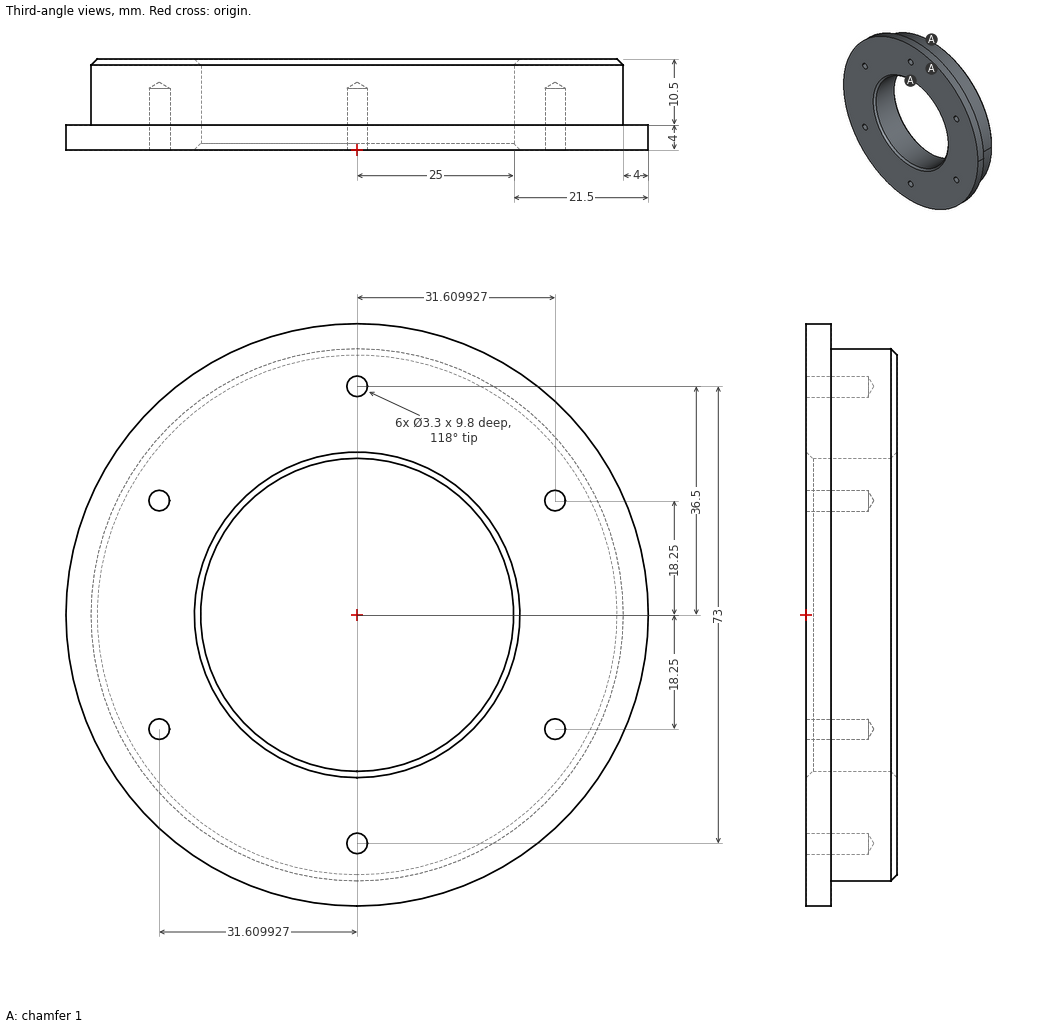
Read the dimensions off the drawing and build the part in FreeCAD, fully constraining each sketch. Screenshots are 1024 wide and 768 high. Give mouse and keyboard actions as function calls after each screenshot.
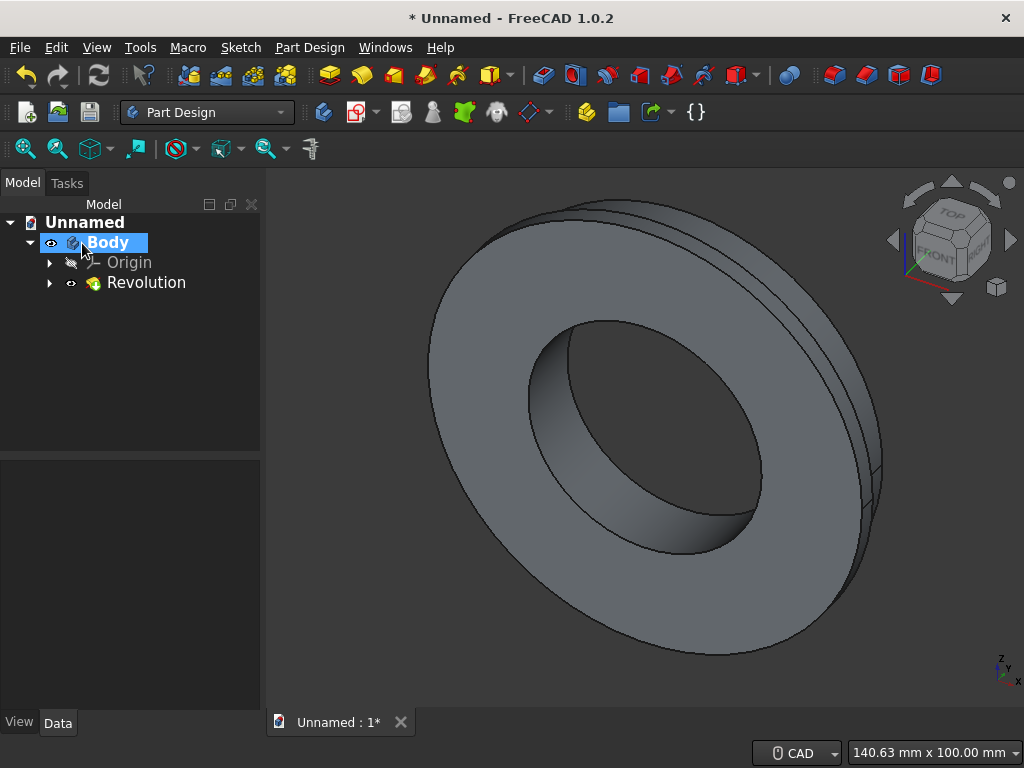
click(26, 150)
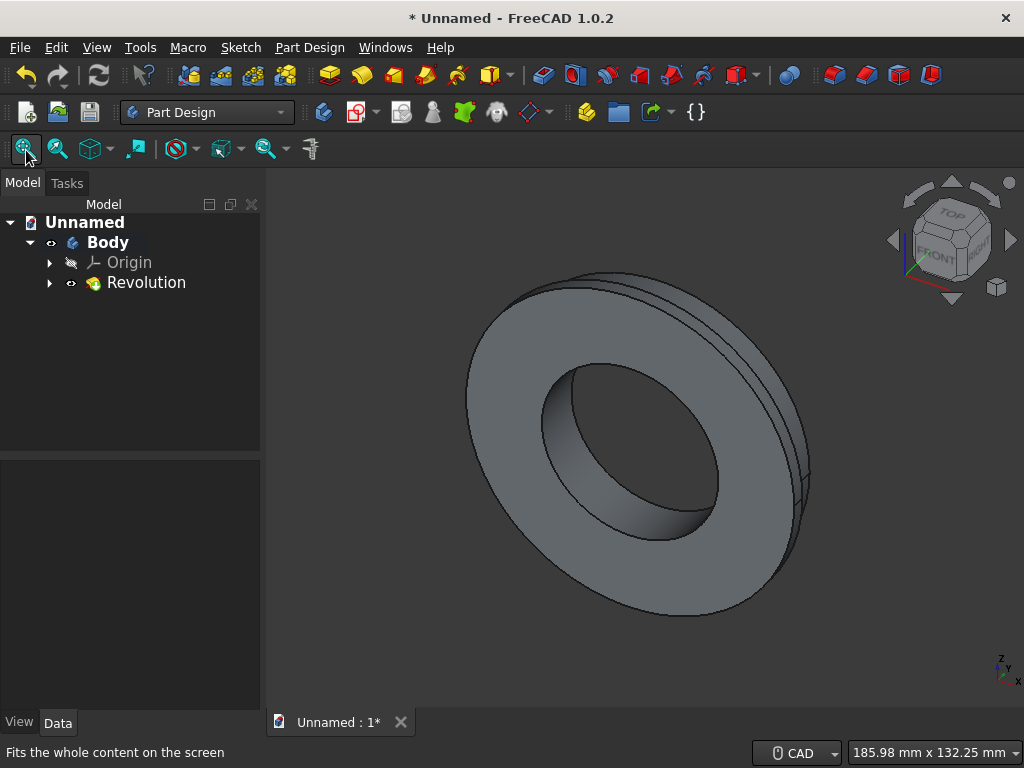
click(536, 509)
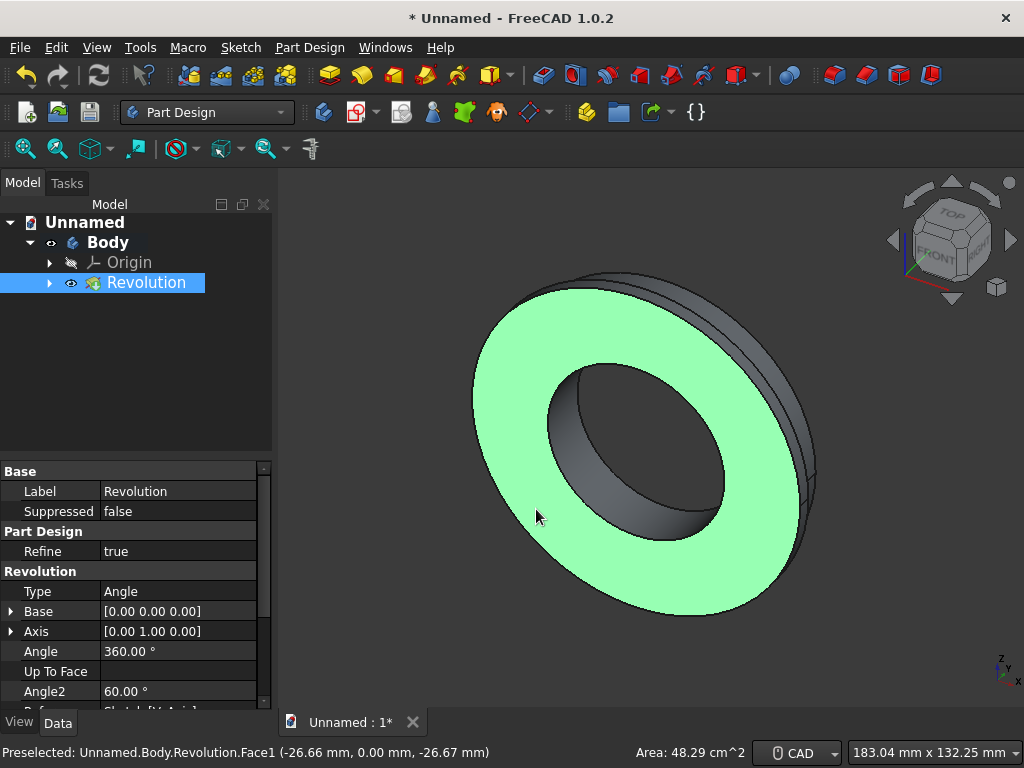
click(356, 112)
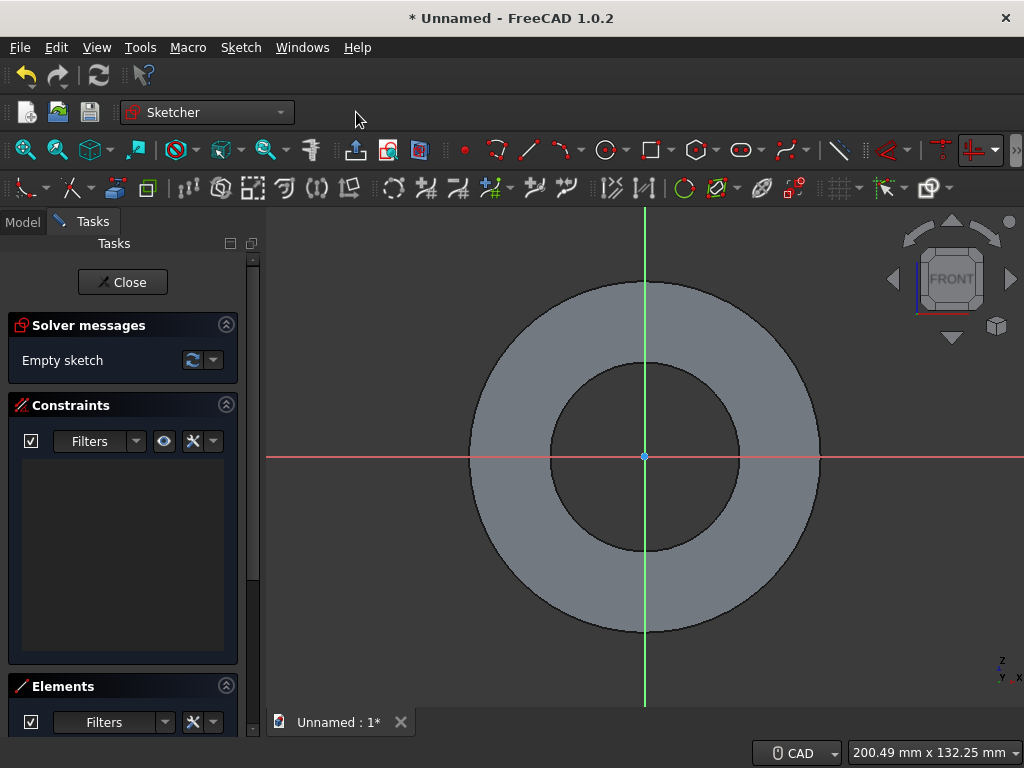
click(606, 150)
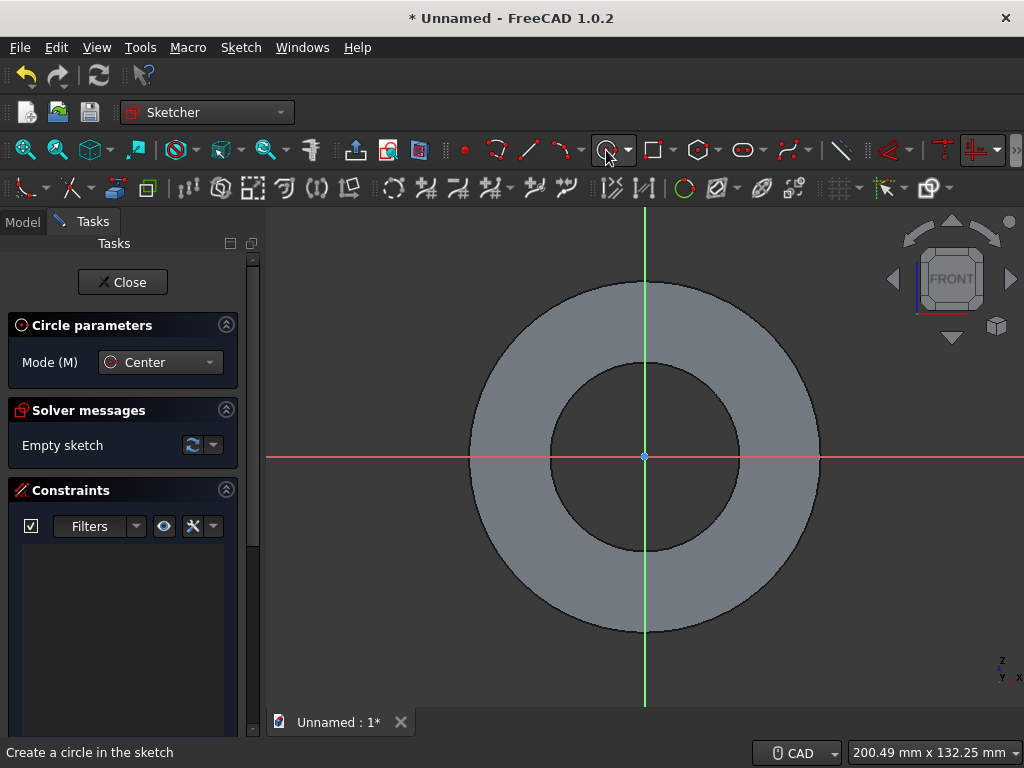
scroll(645, 319, up, 7)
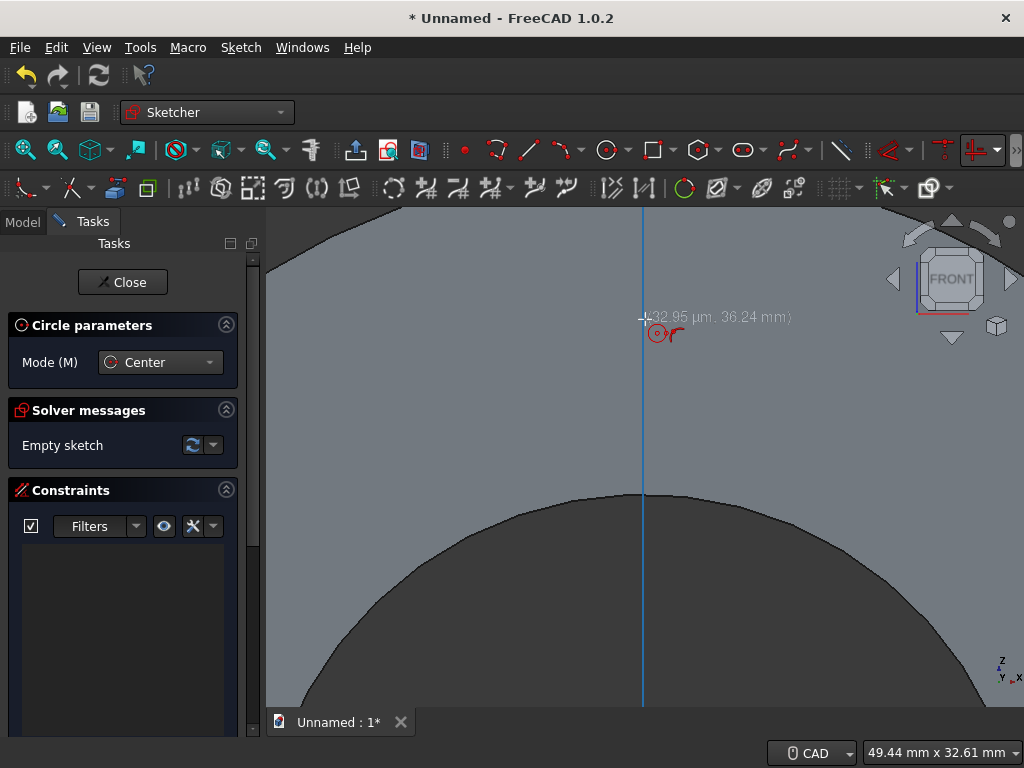
scroll(555, 319, down, 7)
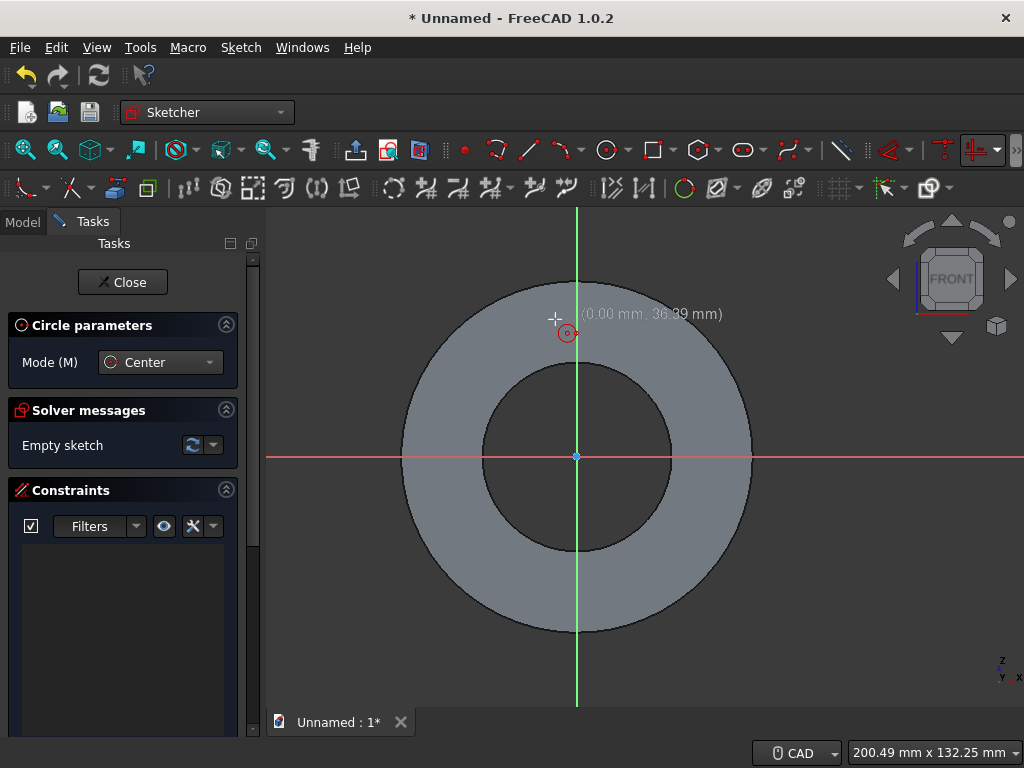
click(577, 319)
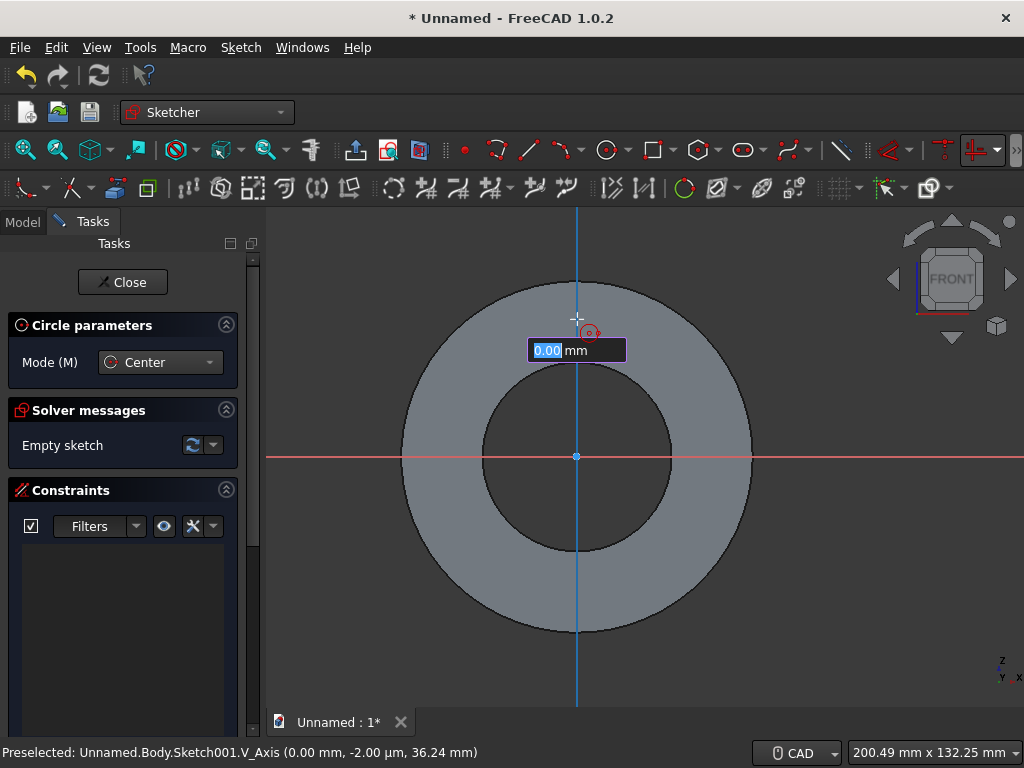
scroll(583, 317, up, 5)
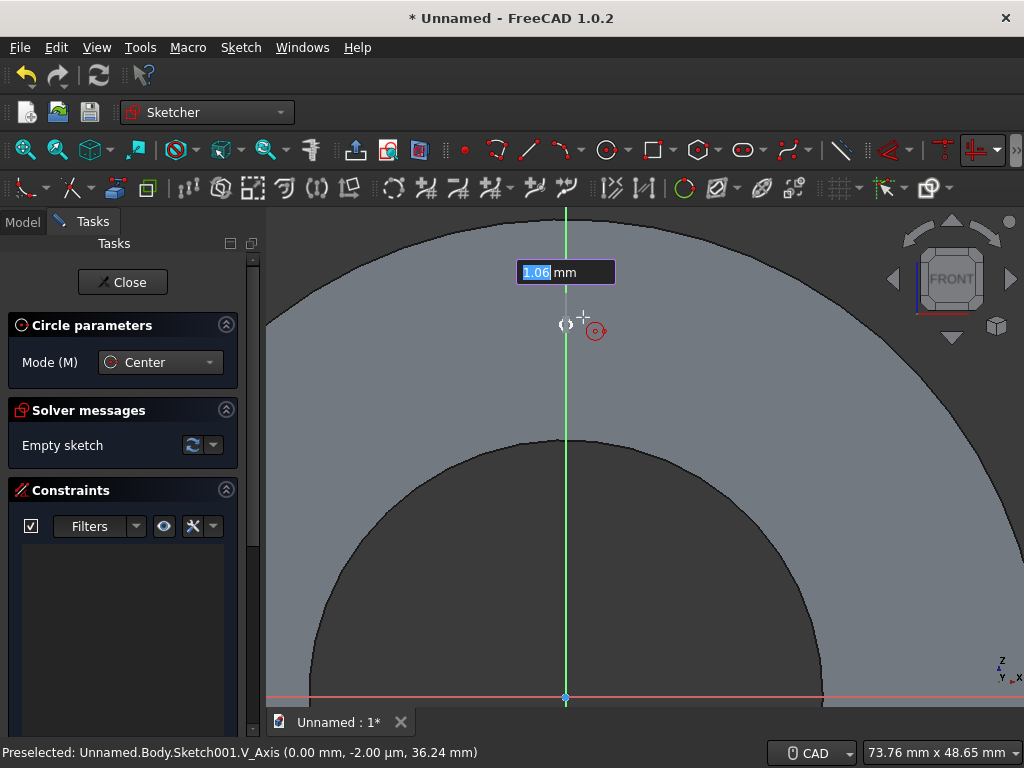
click(582, 316)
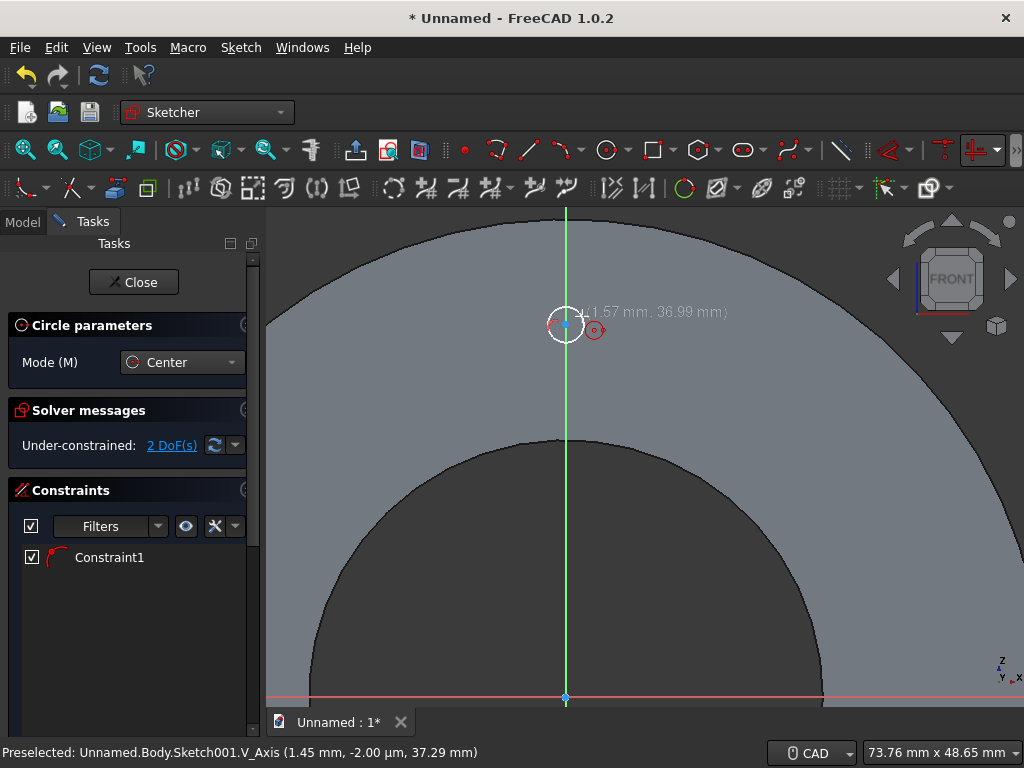
scroll(583, 317, down, 5)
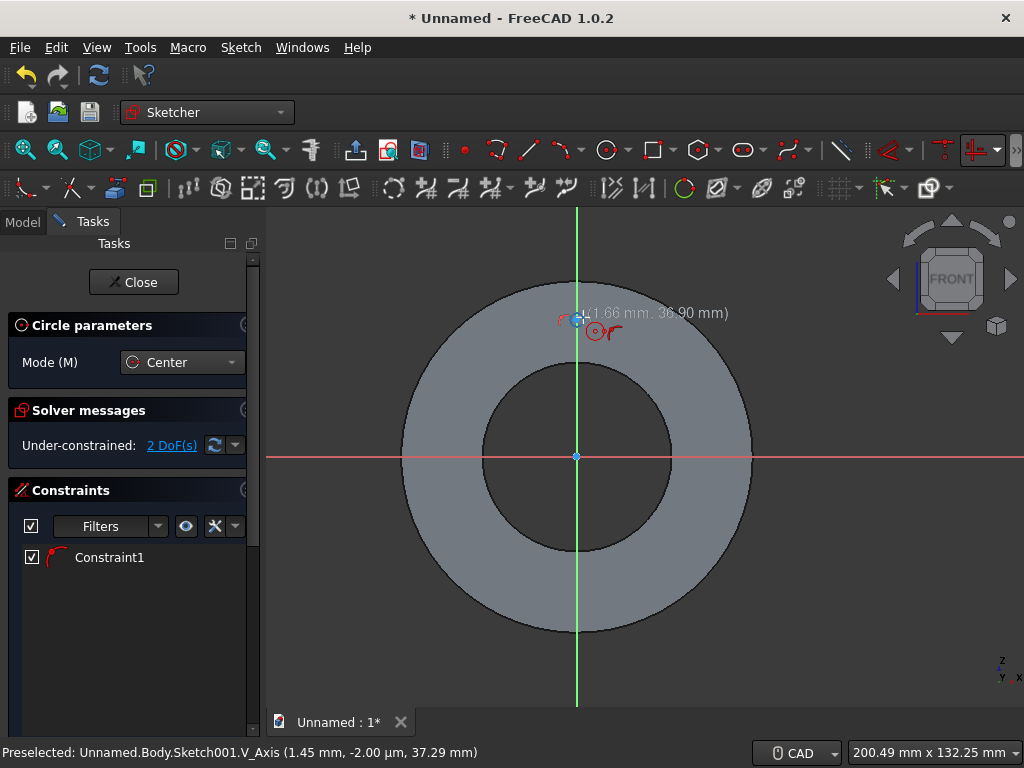
scroll(696, 388, up, 7)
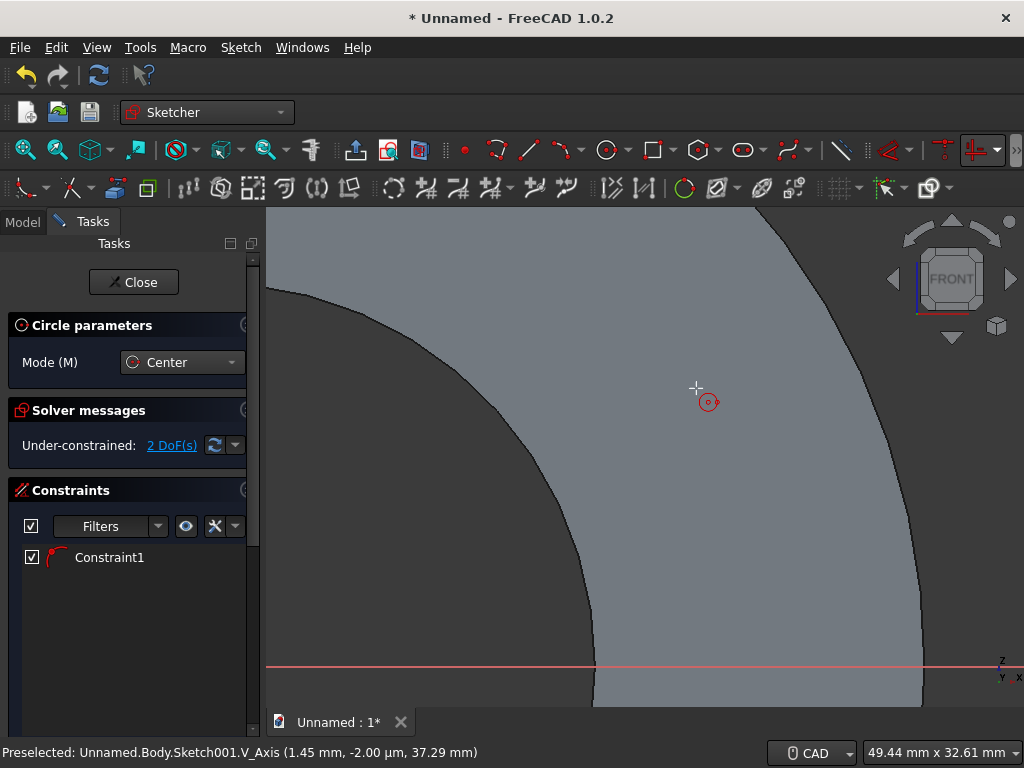
scroll(696, 388, down, 7)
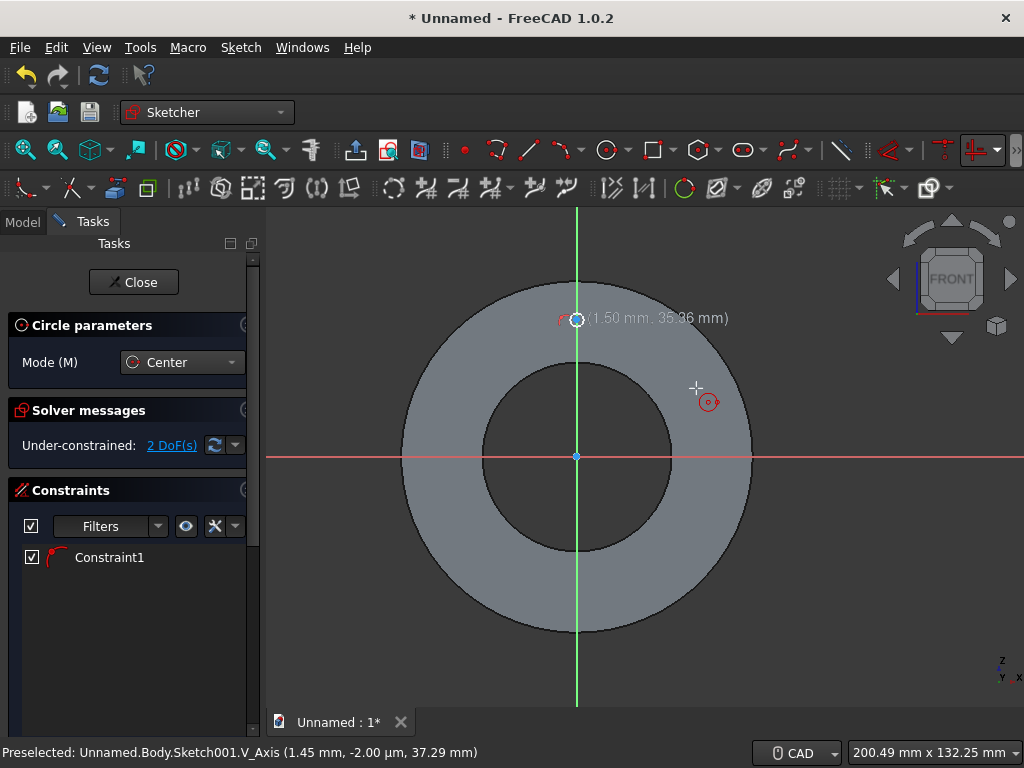
click(696, 388)